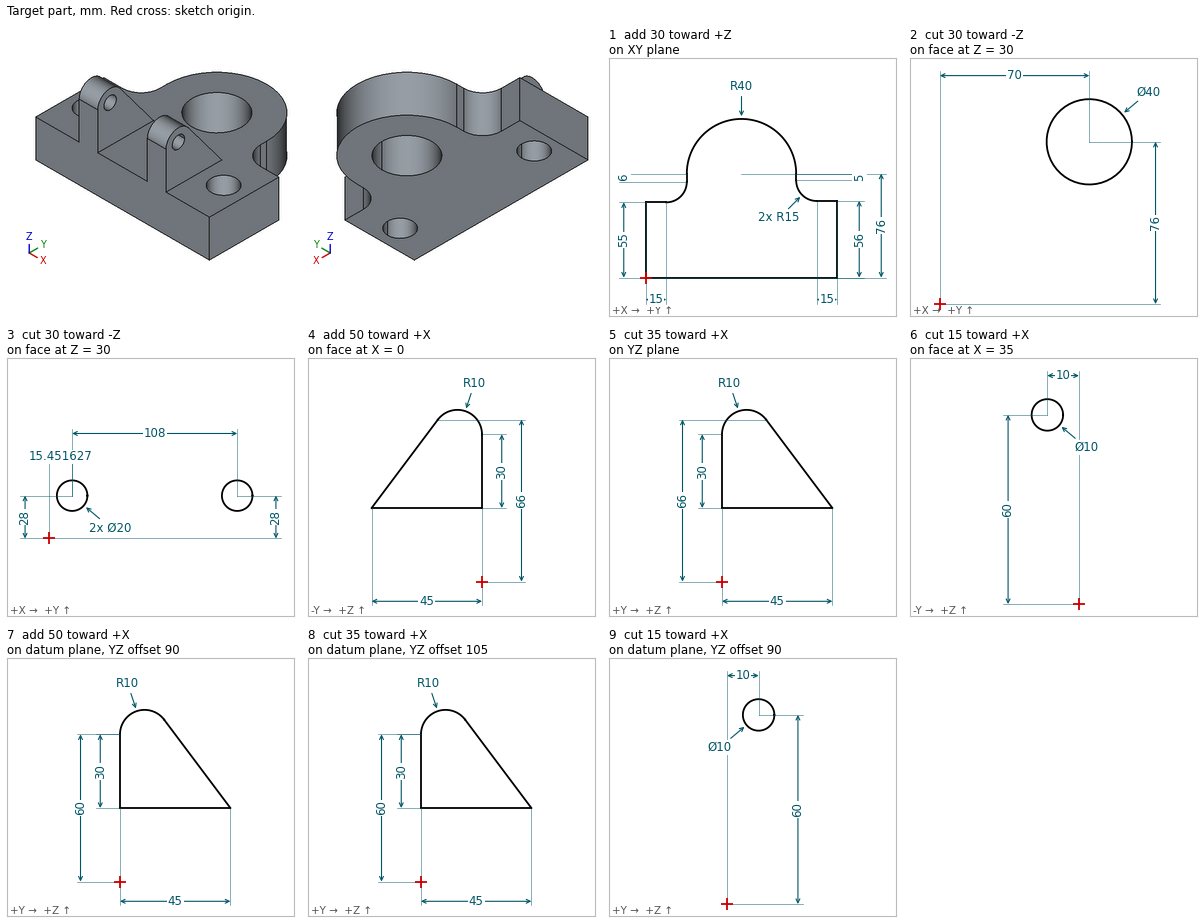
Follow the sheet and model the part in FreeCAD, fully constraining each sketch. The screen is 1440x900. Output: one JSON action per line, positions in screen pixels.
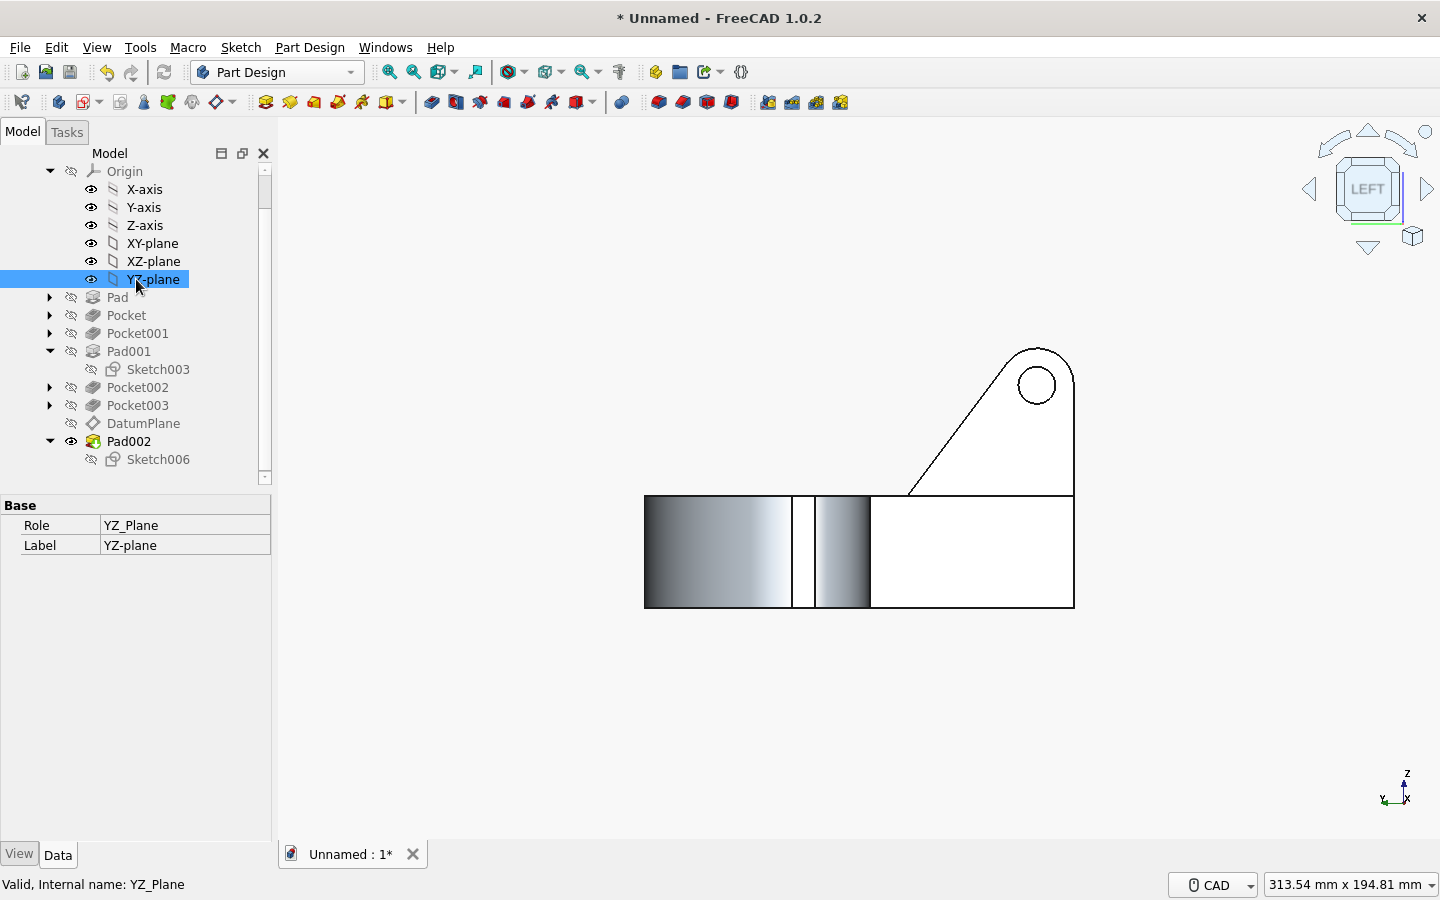
{"action": "left_click", "coordinate": [216, 102]}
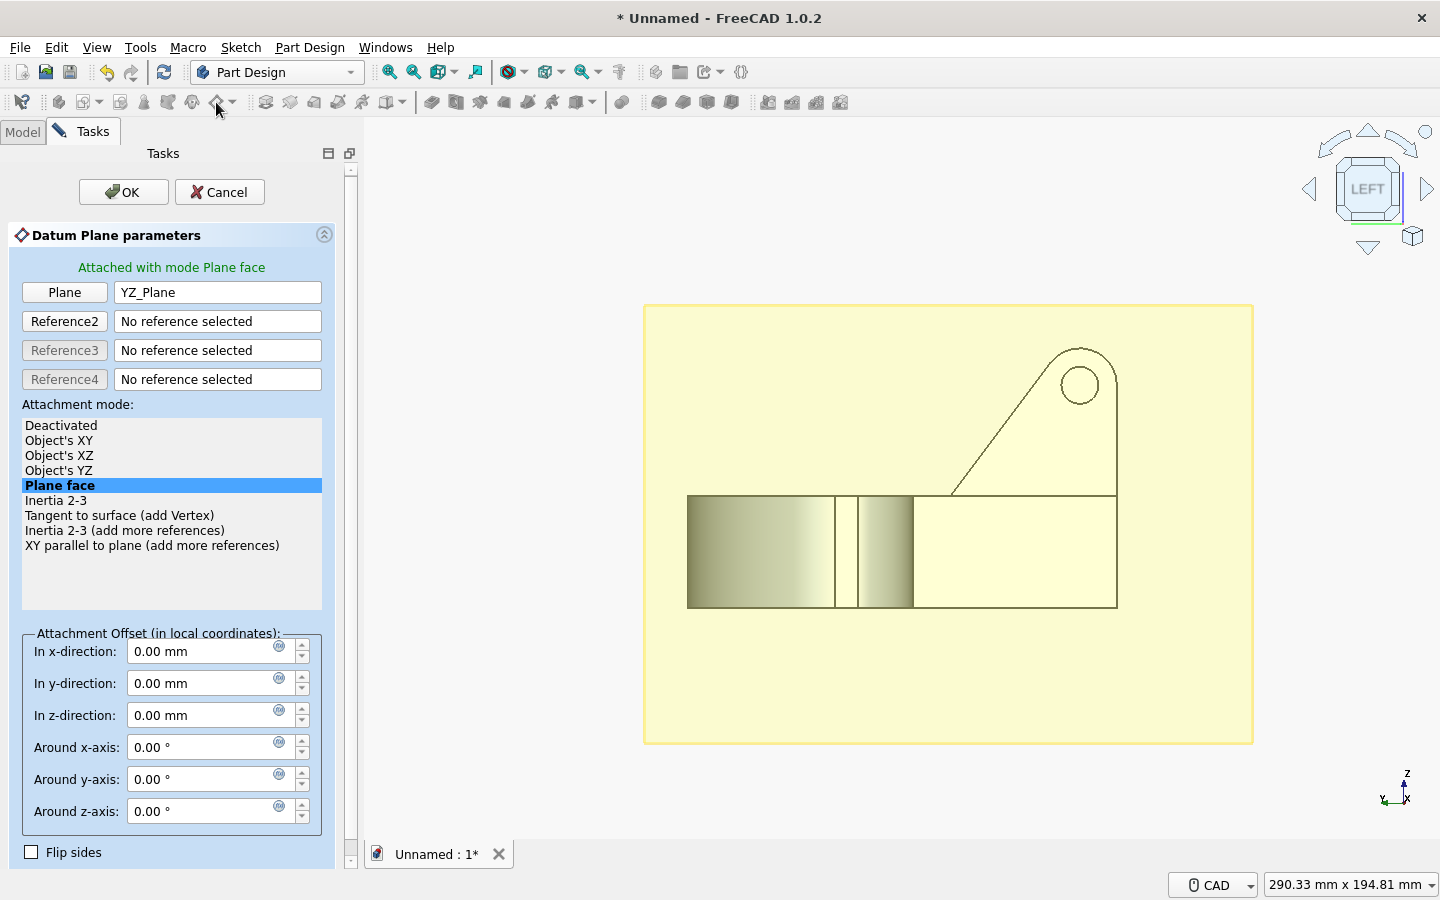
{"action": "triple_click", "coordinate": [210, 715]}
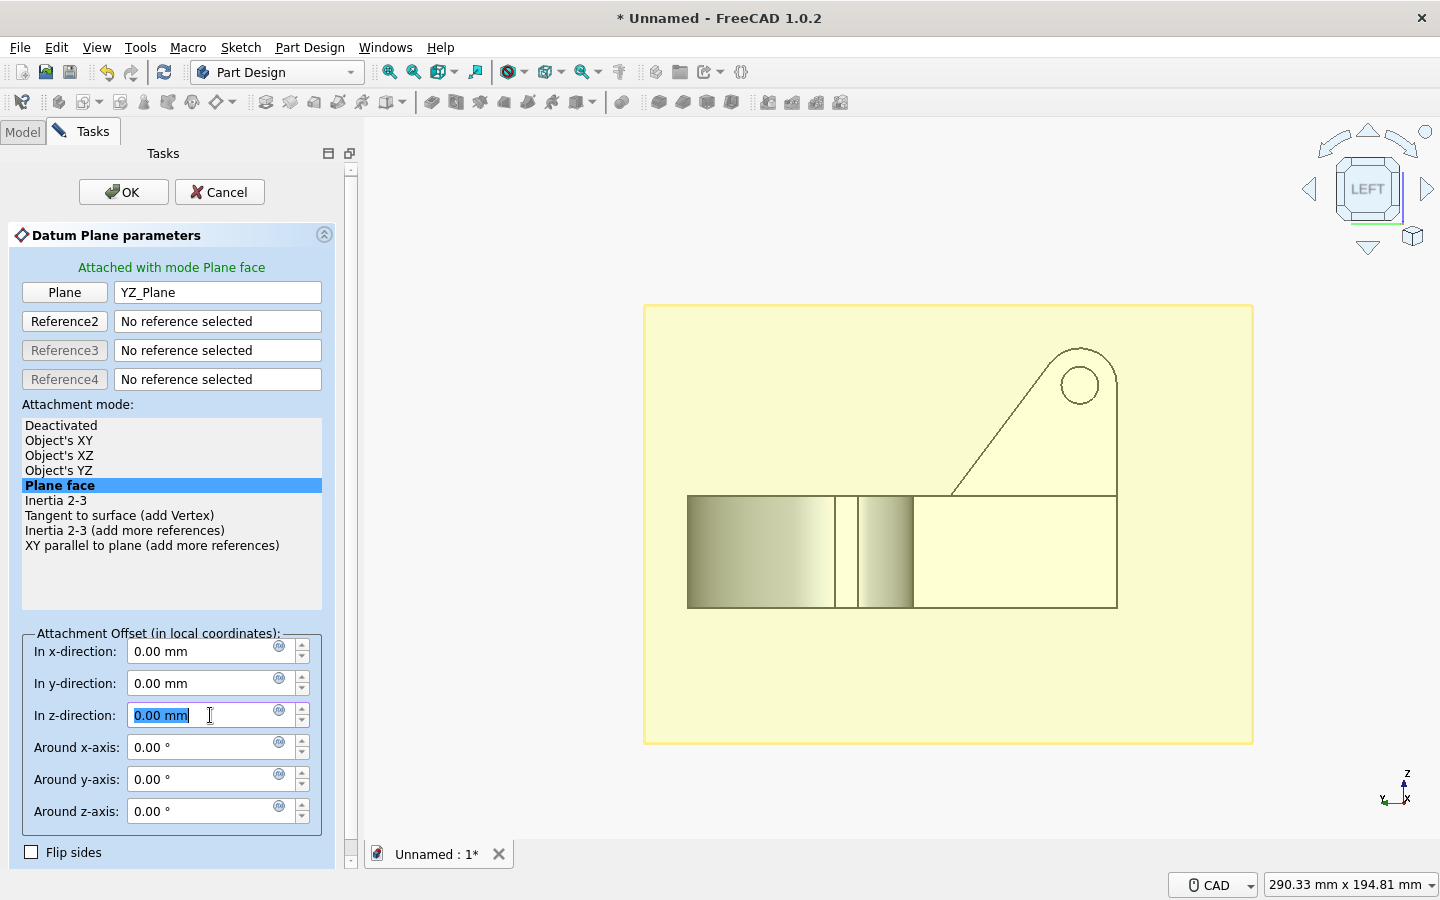
{"action": "type", "text": "105"}
{"action": "key", "text": "Tab"}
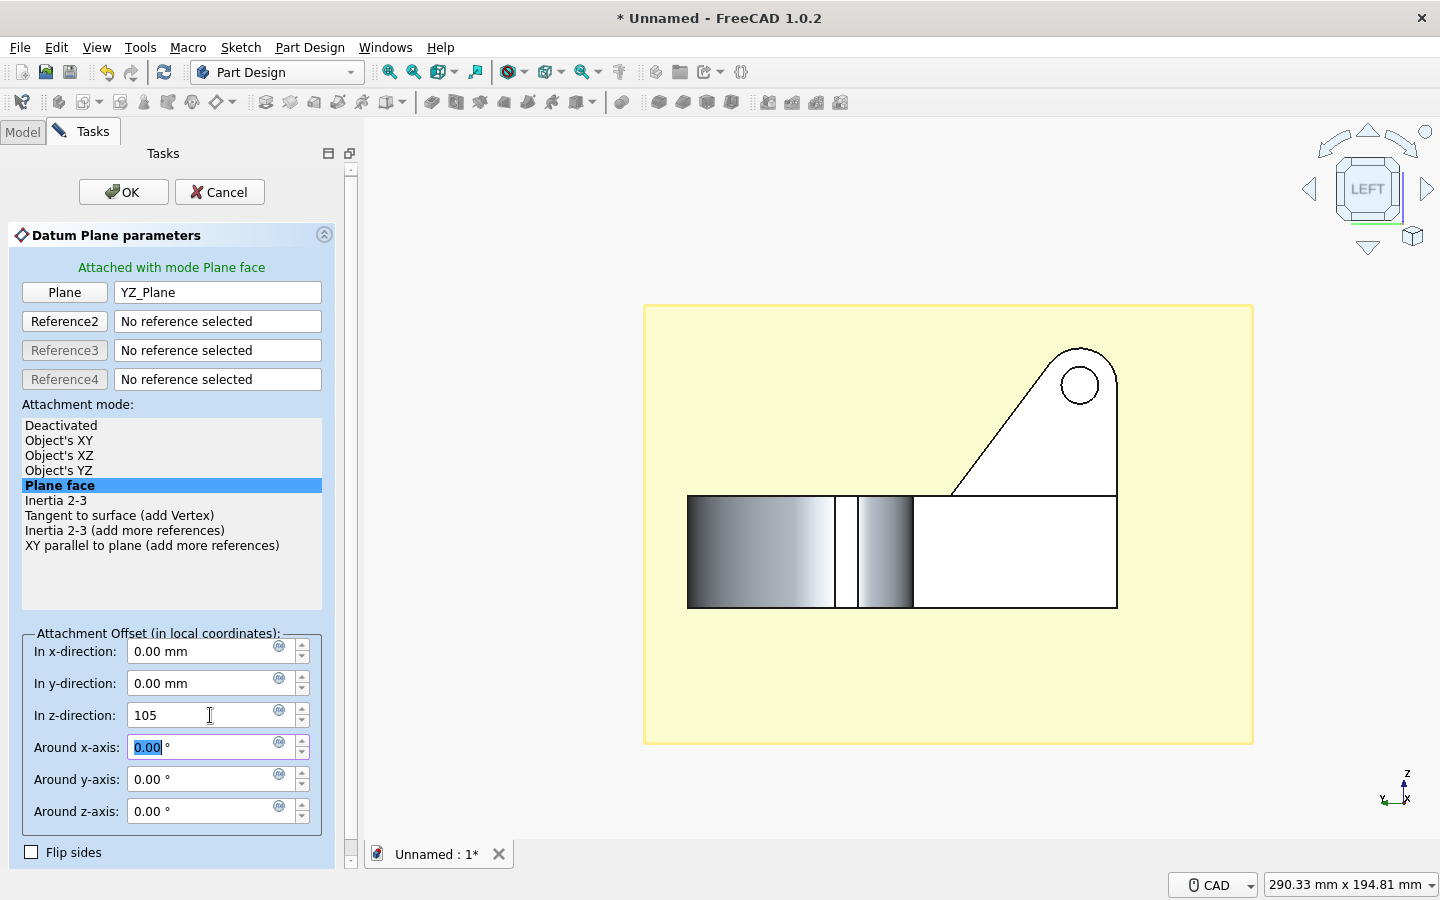
{"action": "left_click", "coordinate": [124, 192]}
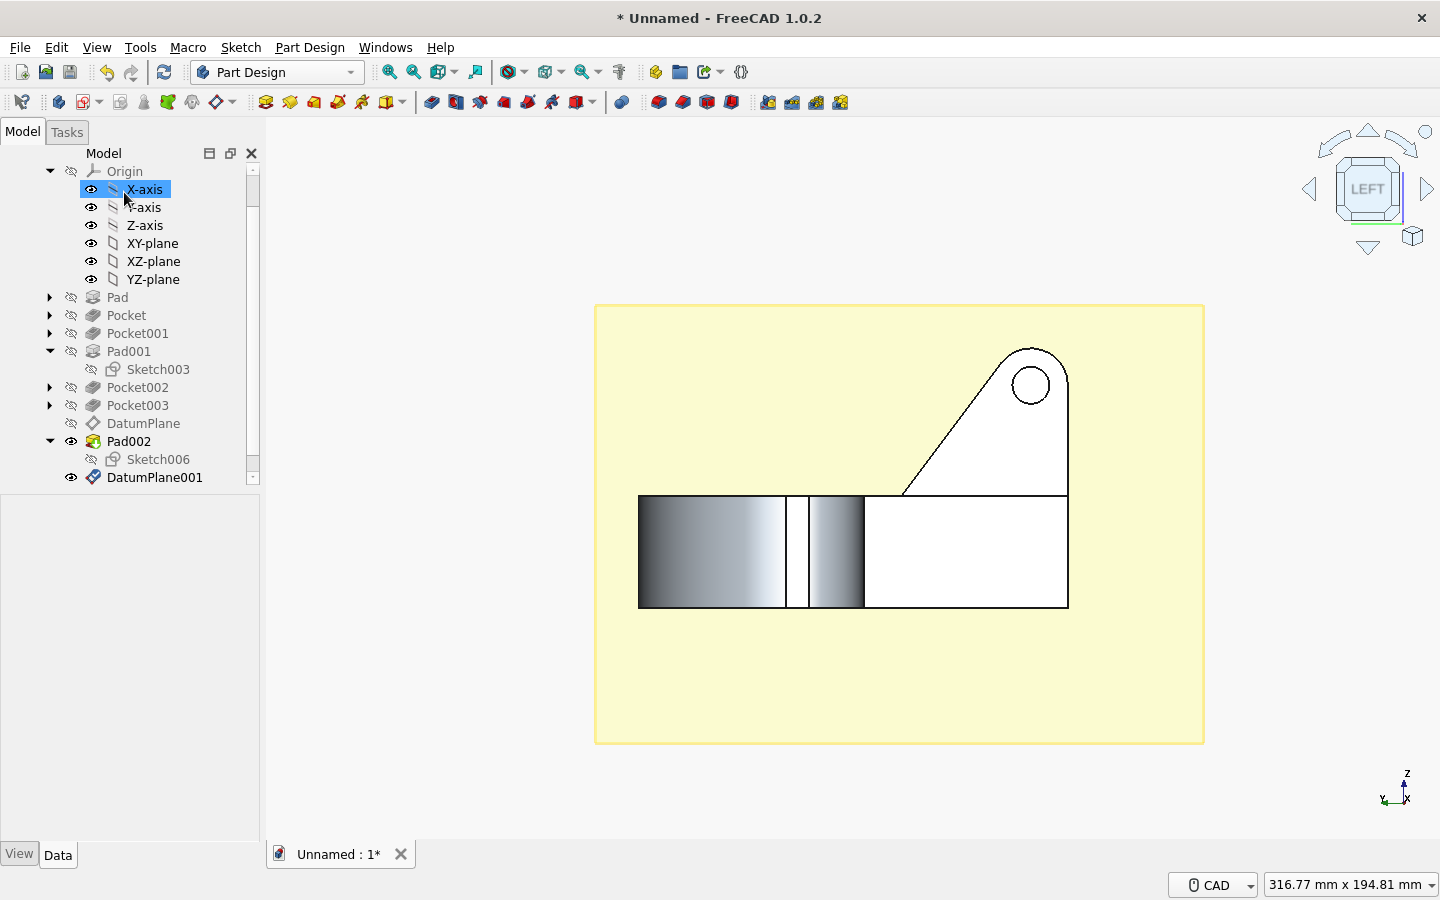
{"action": "left_click", "coordinate": [116, 477]}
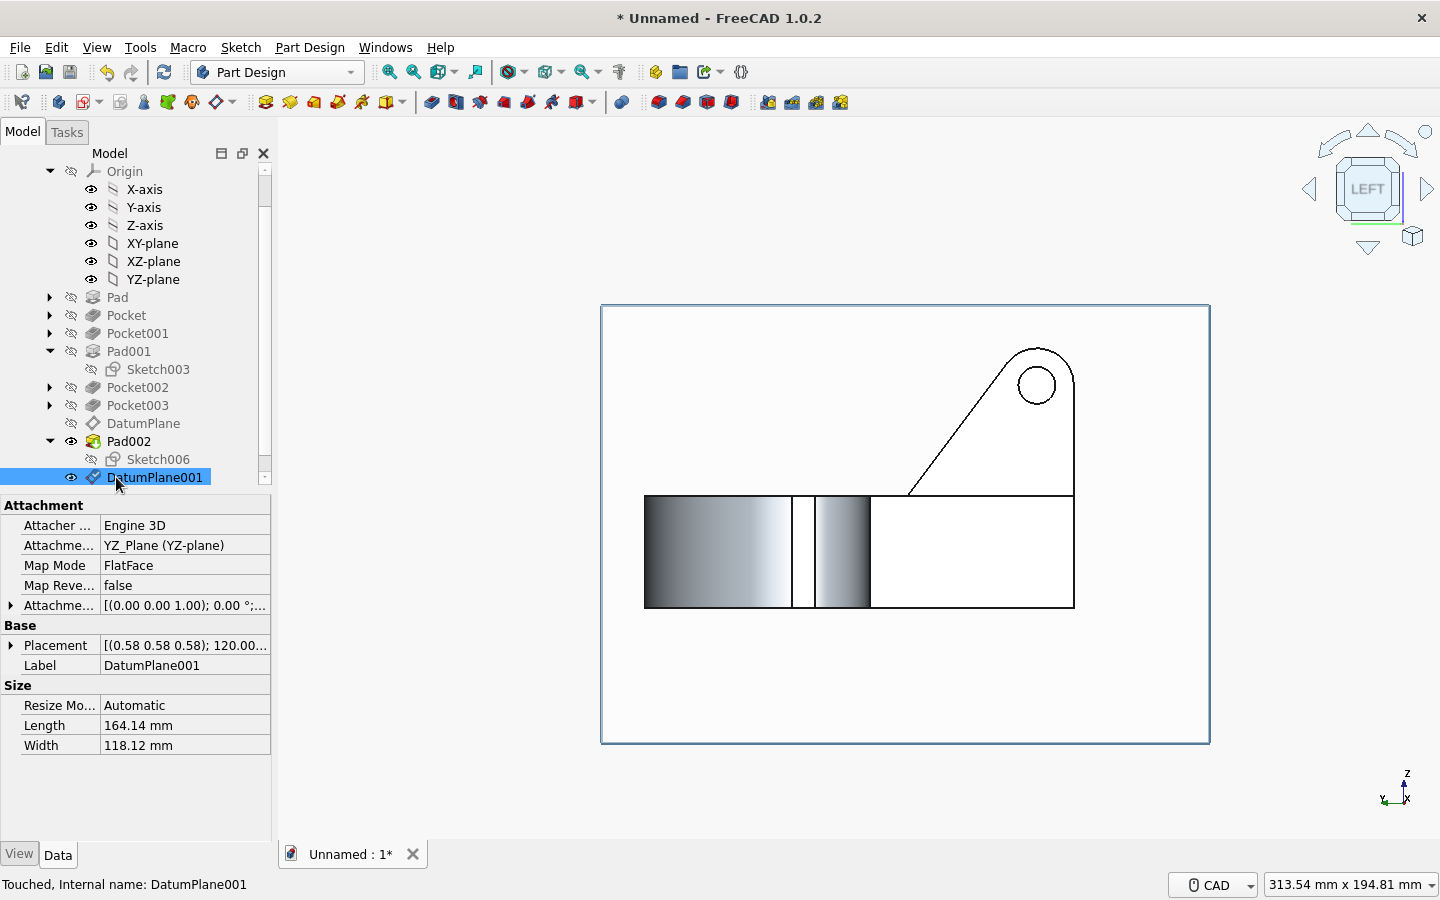
{"action": "left_click", "coordinate": [84, 102]}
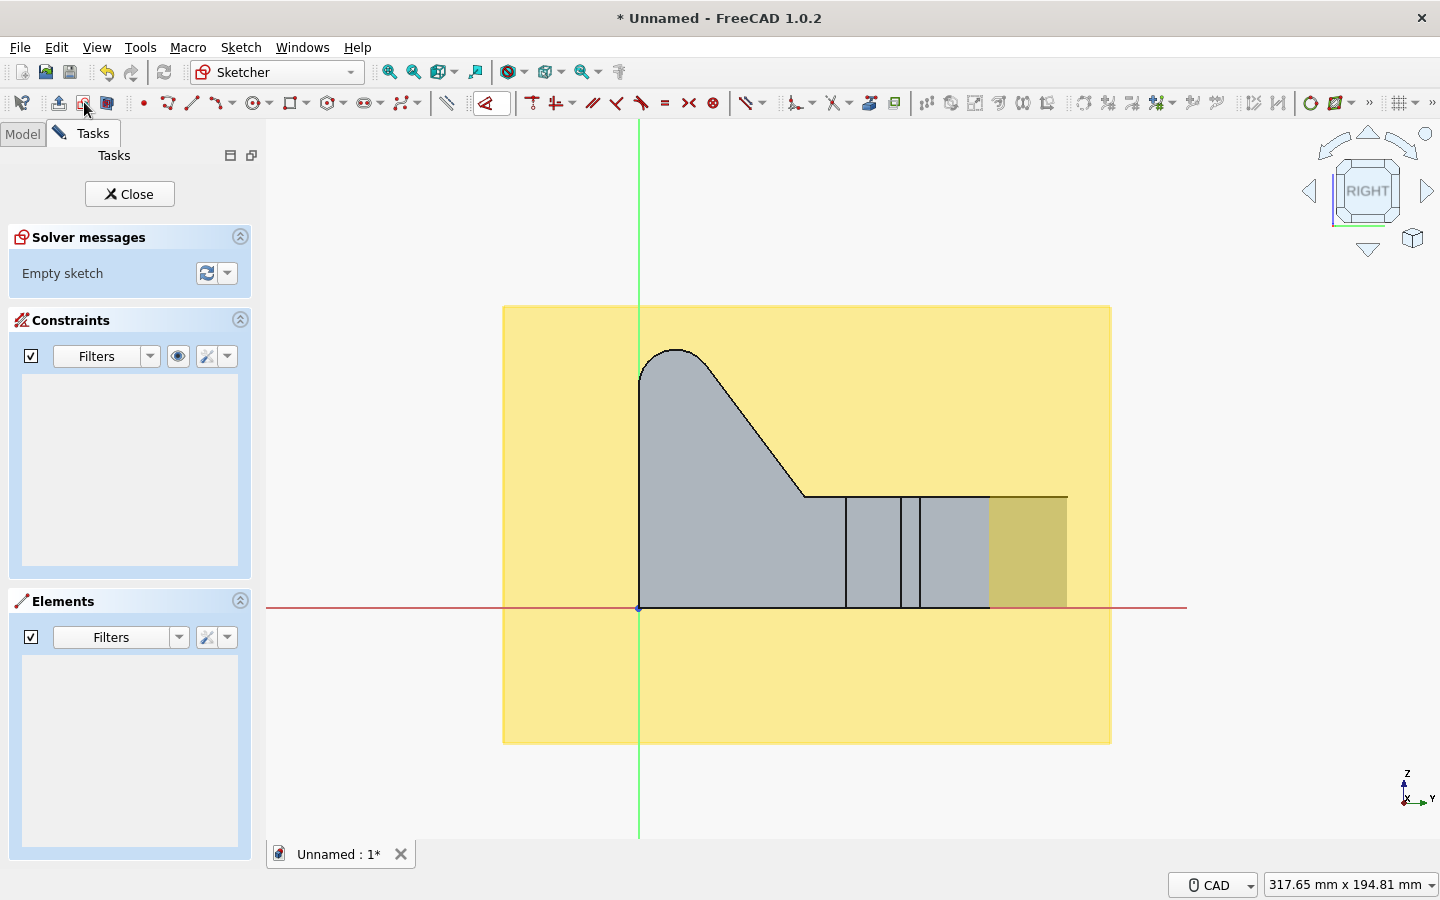
{"action": "left_click", "coordinate": [108, 104]}